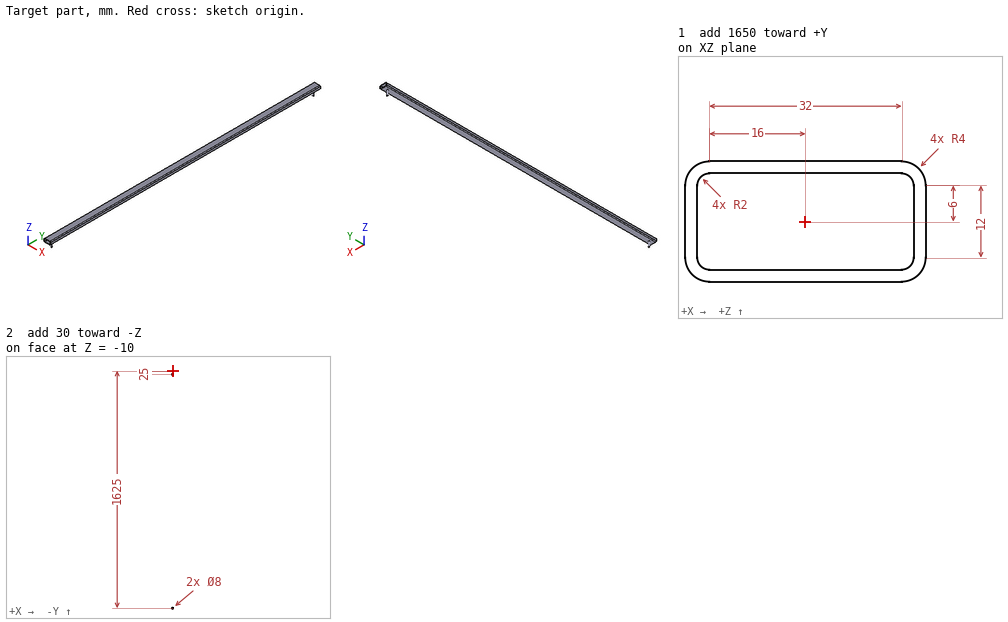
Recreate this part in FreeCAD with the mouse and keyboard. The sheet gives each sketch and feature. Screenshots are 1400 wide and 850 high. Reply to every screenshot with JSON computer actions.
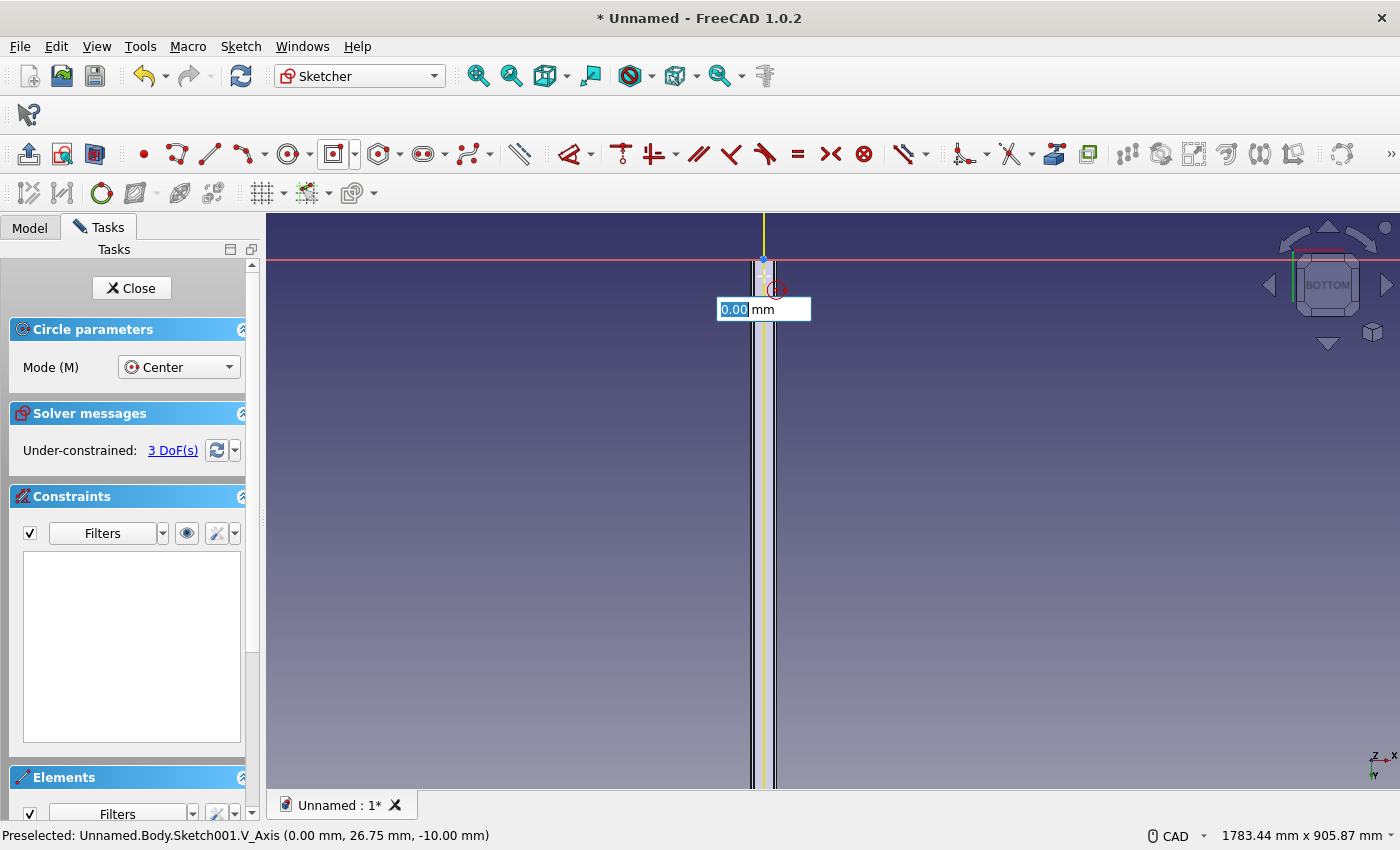
{"action": "scroll", "coordinate": [766, 275], "scroll_direction": "up", "scroll_amount": 10}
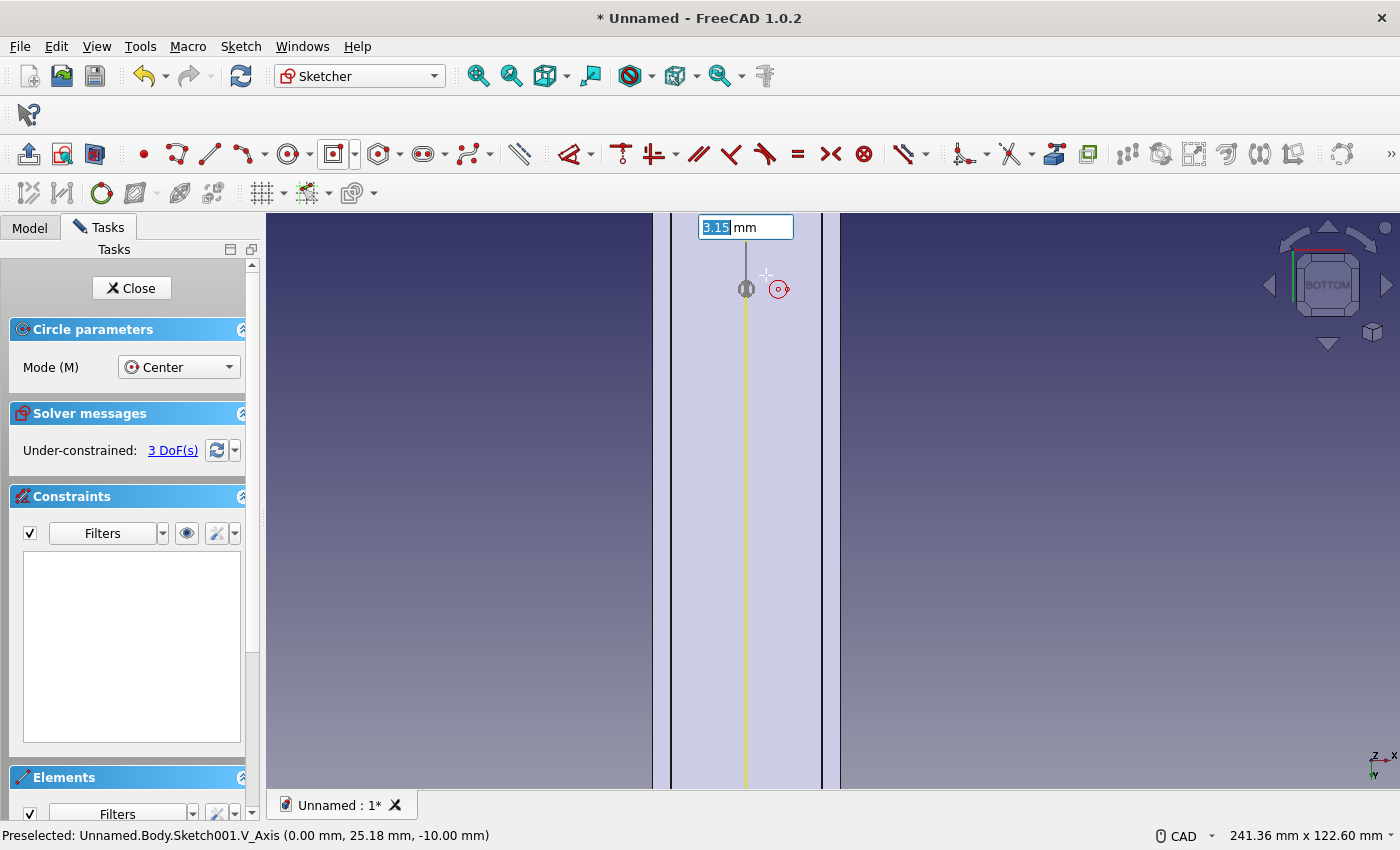
{"action": "left_click", "coordinate": [764, 274]}
{"action": "key", "text": "Escape"}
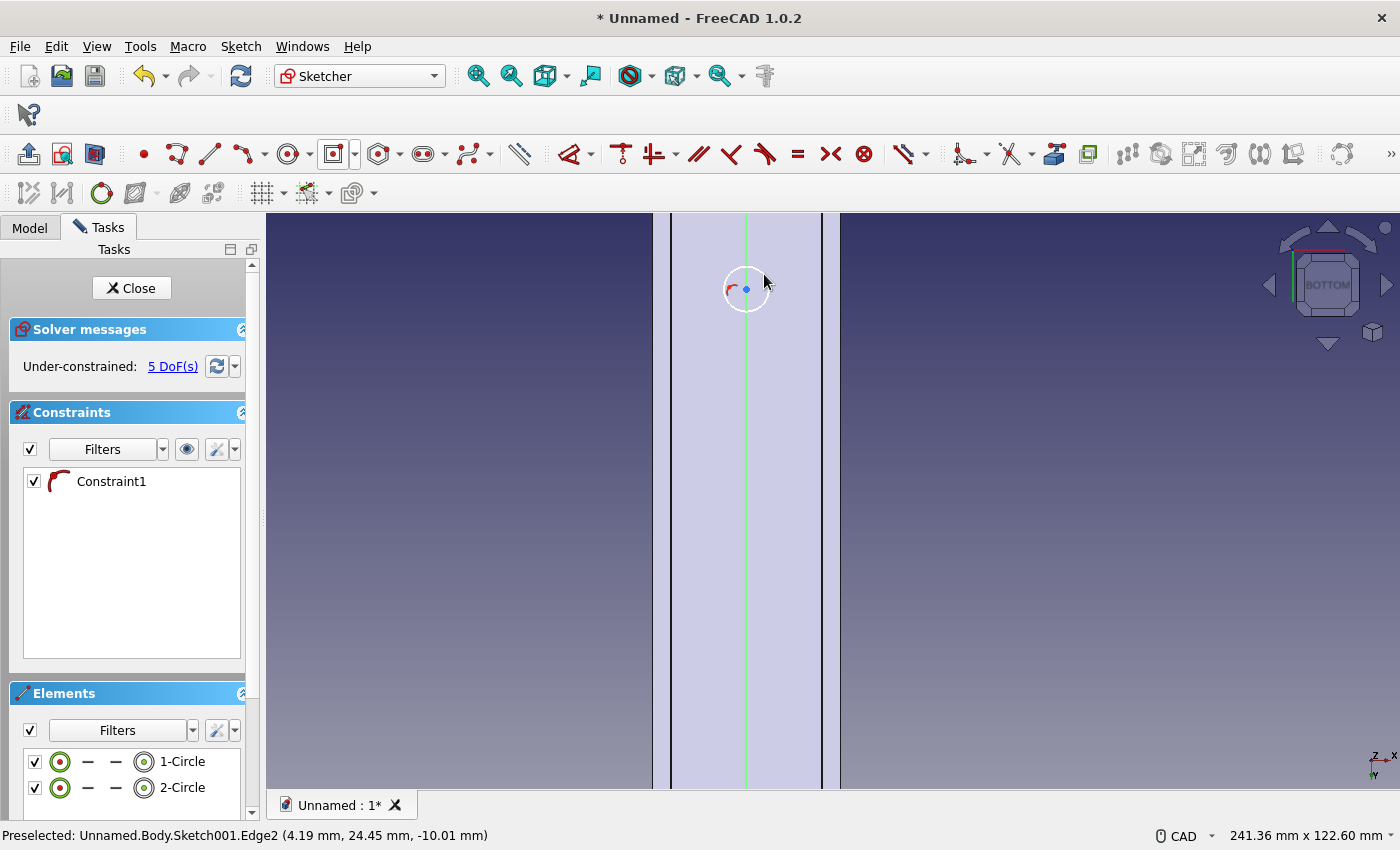
{"action": "scroll", "coordinate": [765, 318], "scroll_direction": "down", "scroll_amount": 15}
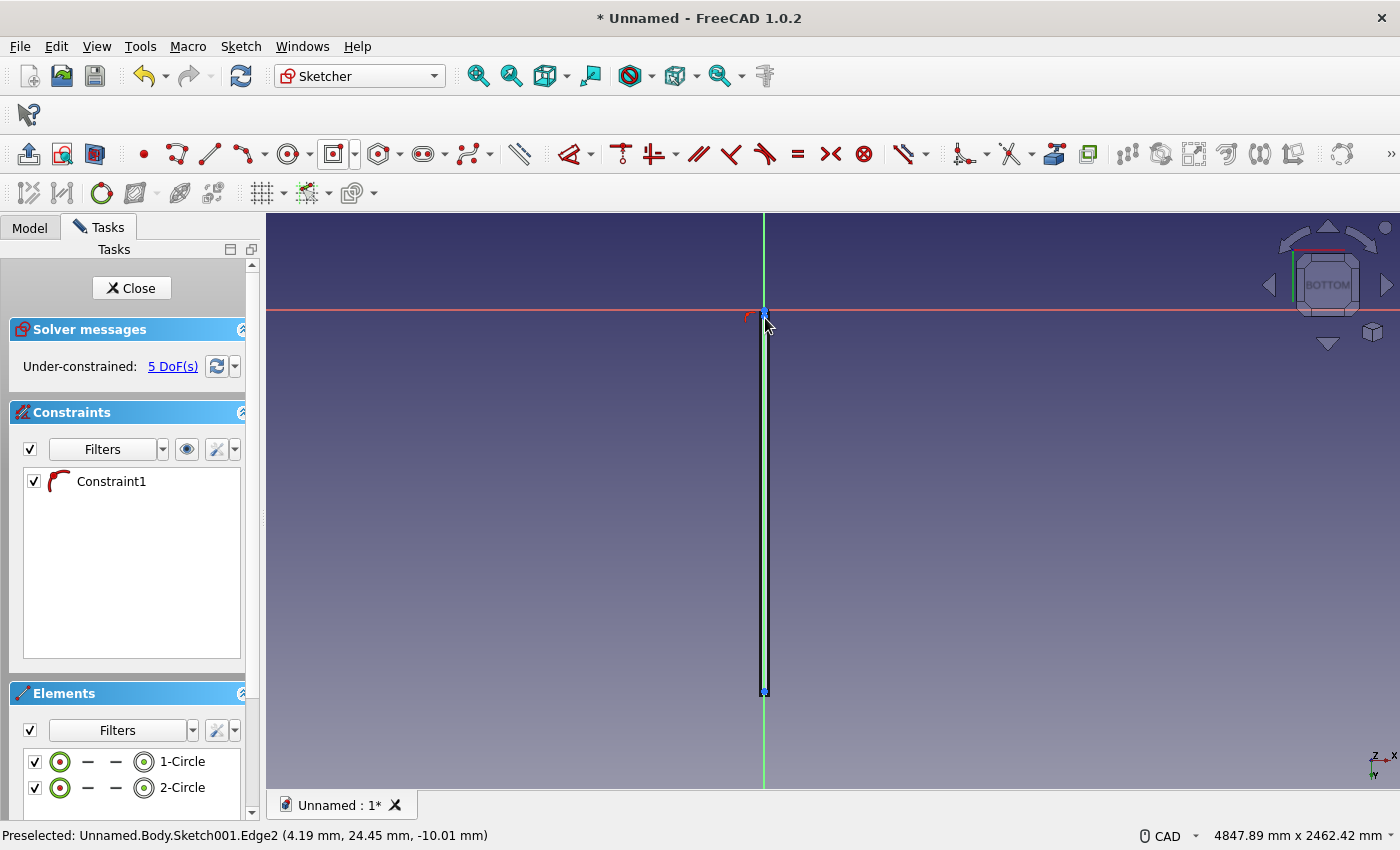
{"action": "scroll", "coordinate": [765, 690], "scroll_direction": "up", "scroll_amount": 14}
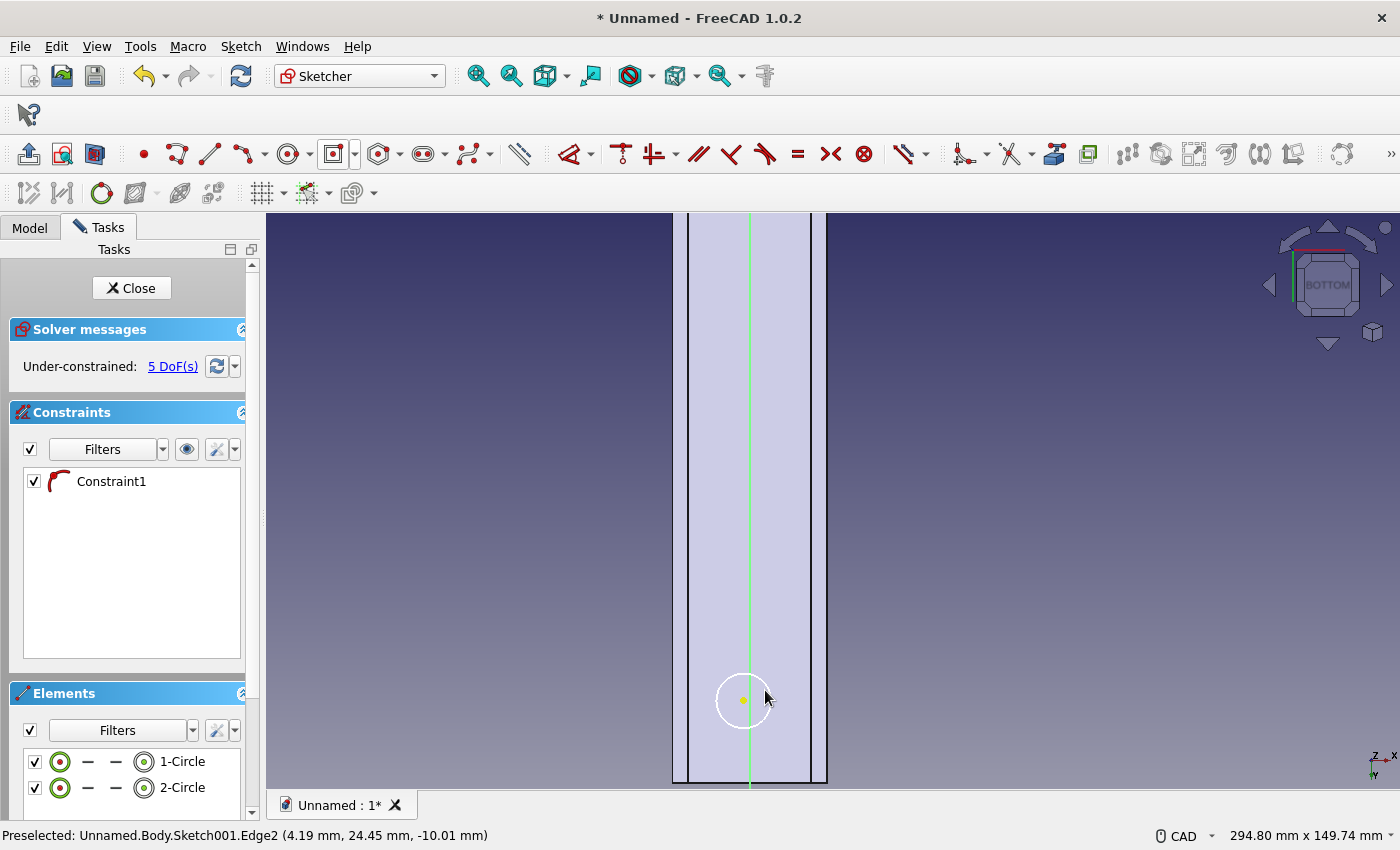
{"action": "left_click", "coordinate": [763, 681]}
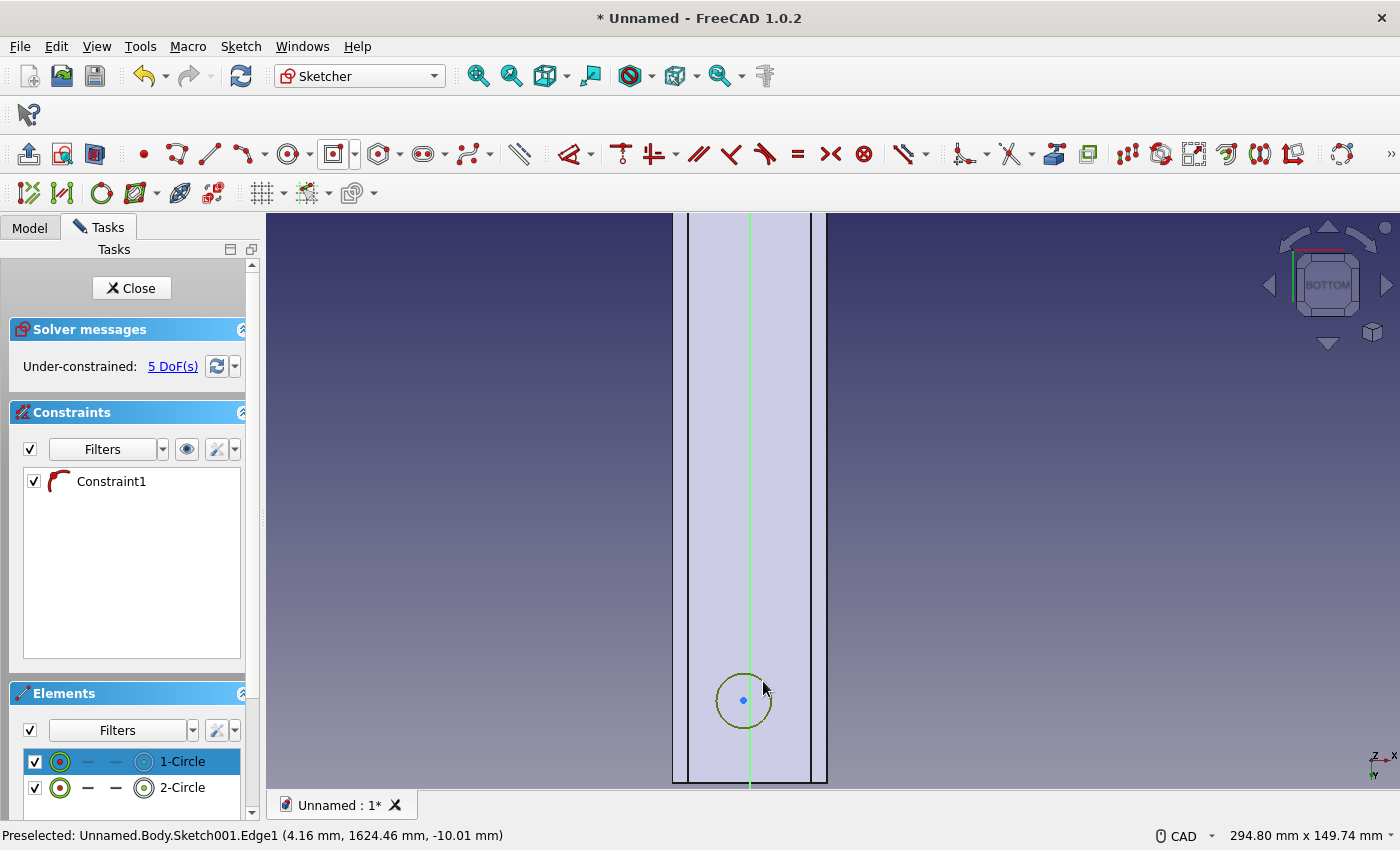
{"action": "scroll", "coordinate": [765, 691], "scroll_direction": "down", "scroll_amount": 14}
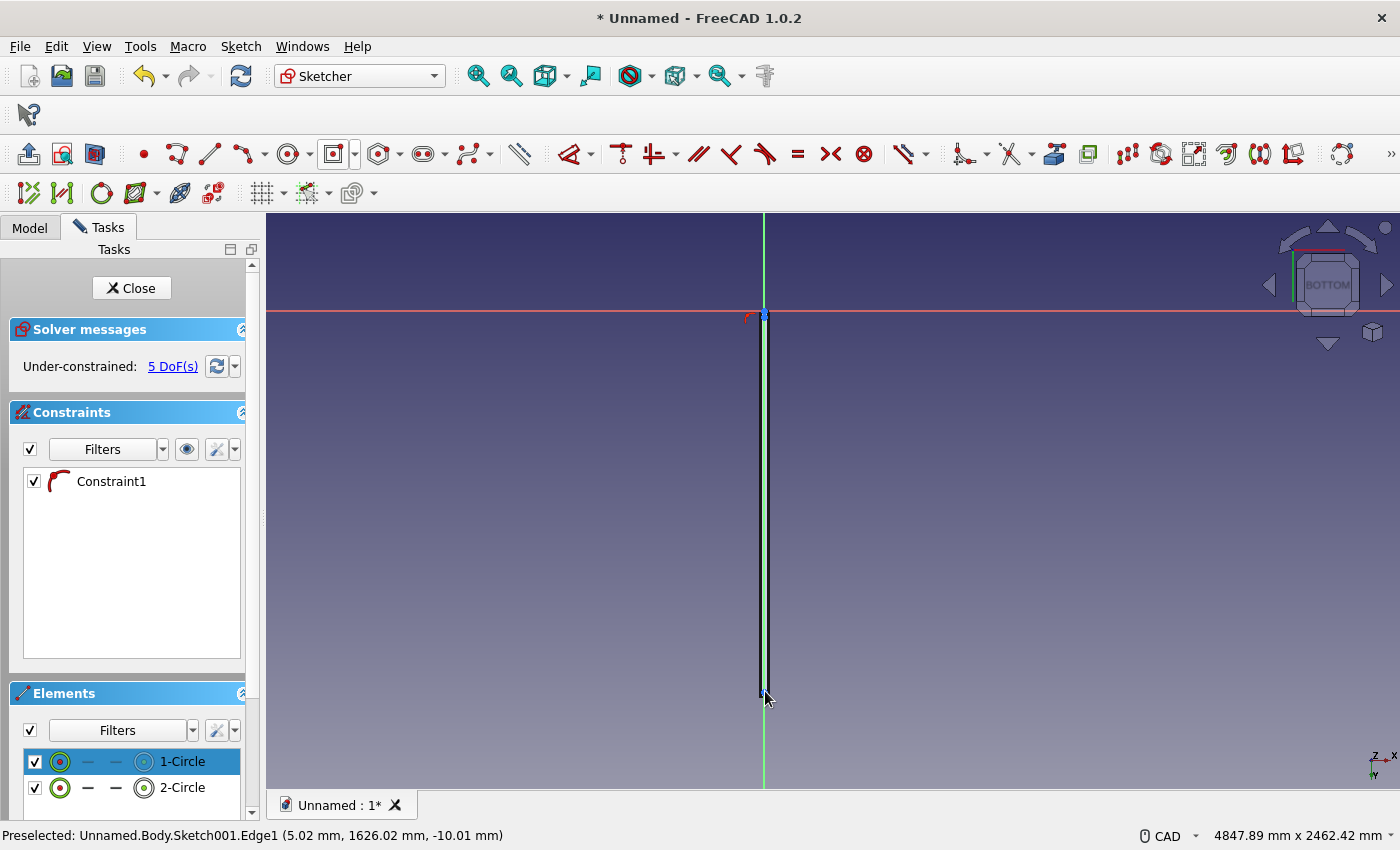
{"action": "scroll", "coordinate": [765, 317], "scroll_direction": "up", "scroll_amount": 14}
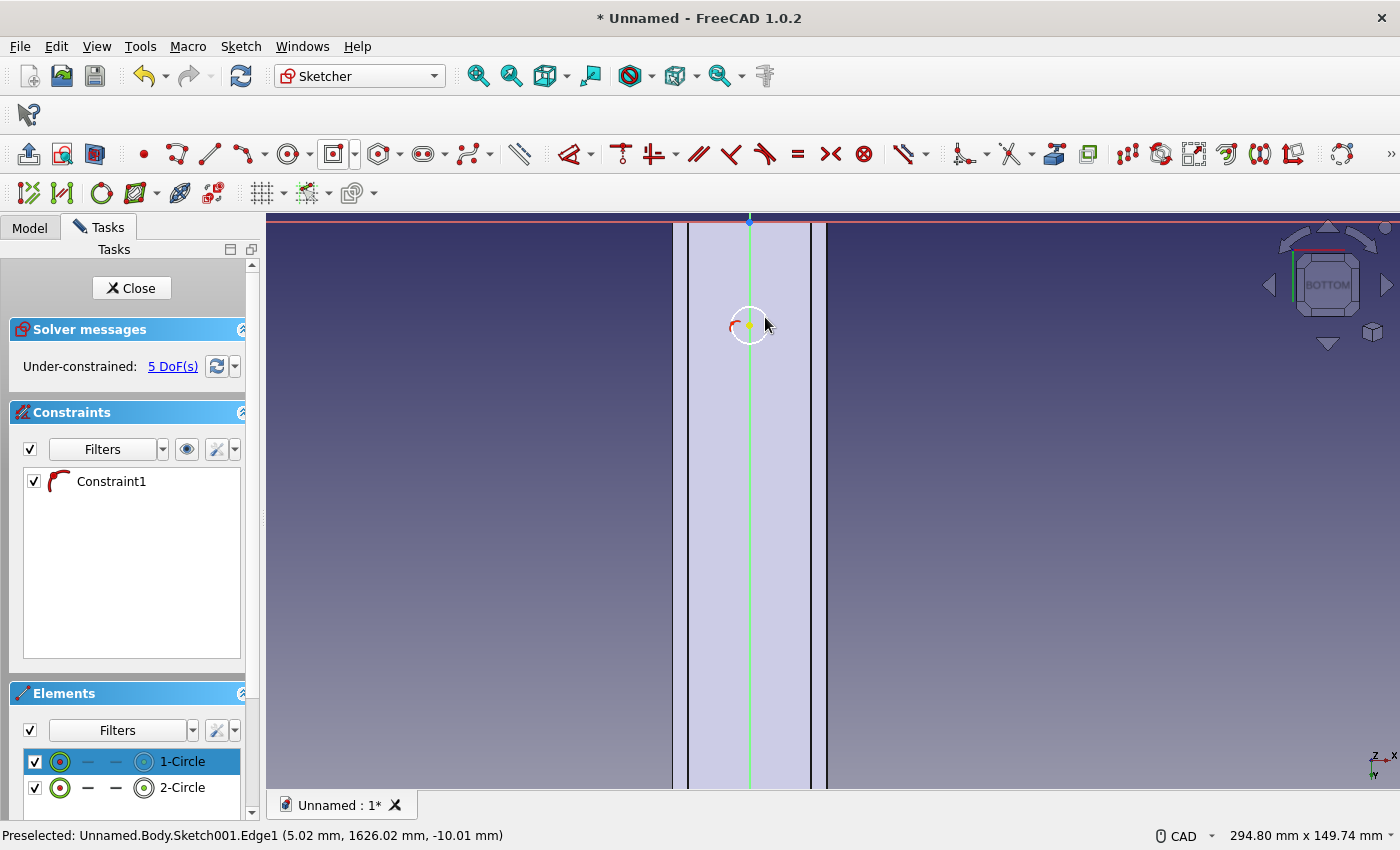
{"action": "left_click", "coordinate": [763, 312]}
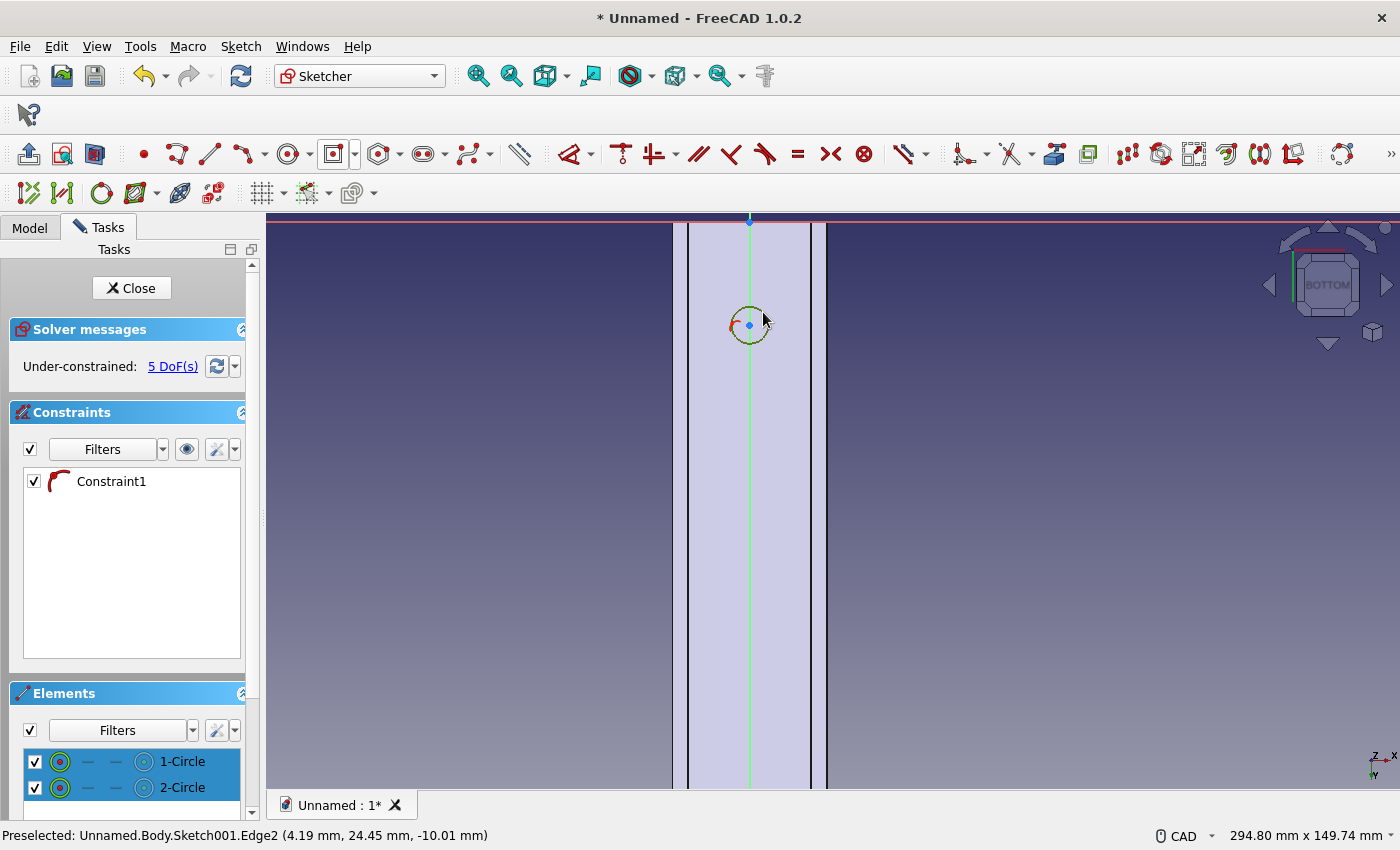
{"action": "key", "text": "e"}